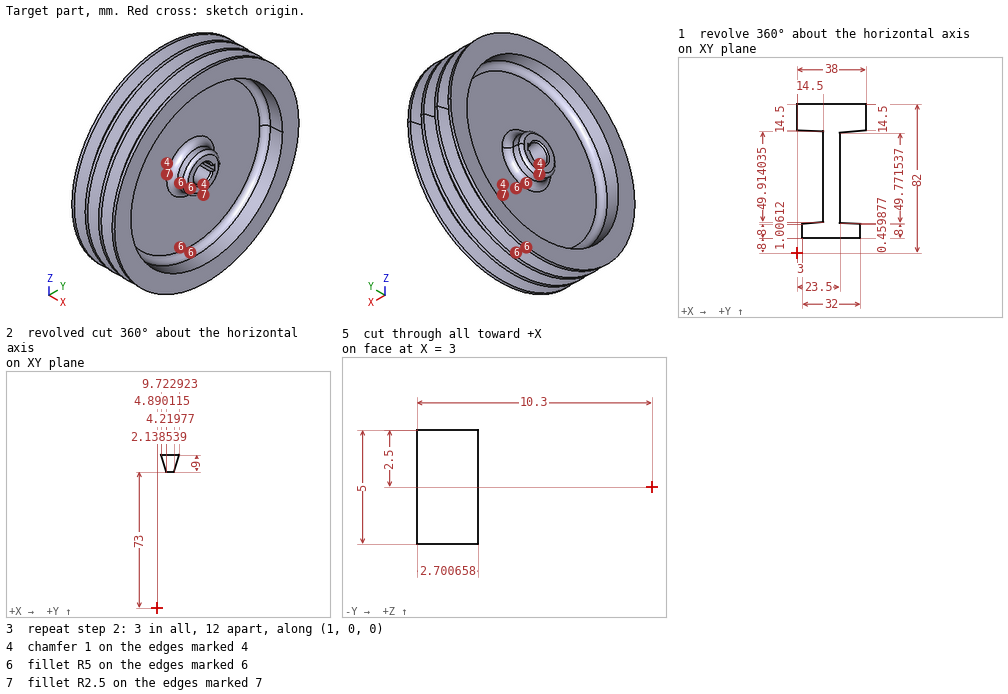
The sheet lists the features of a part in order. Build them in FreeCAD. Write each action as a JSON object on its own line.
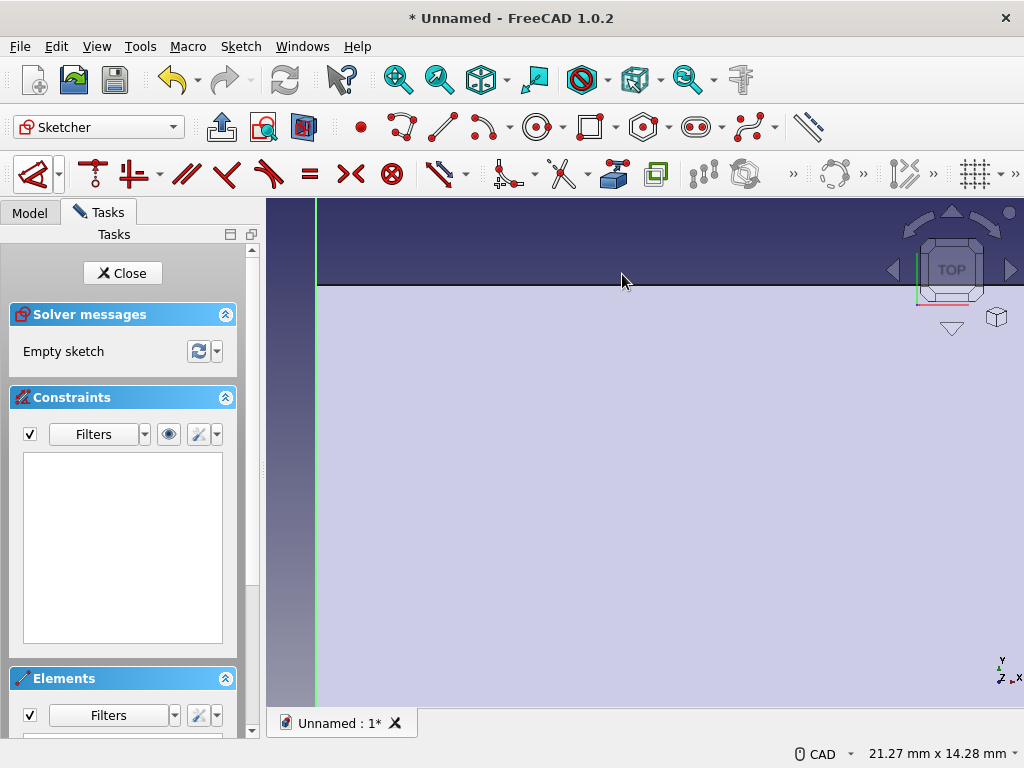
{"action": "left_click", "coordinate": [402, 128]}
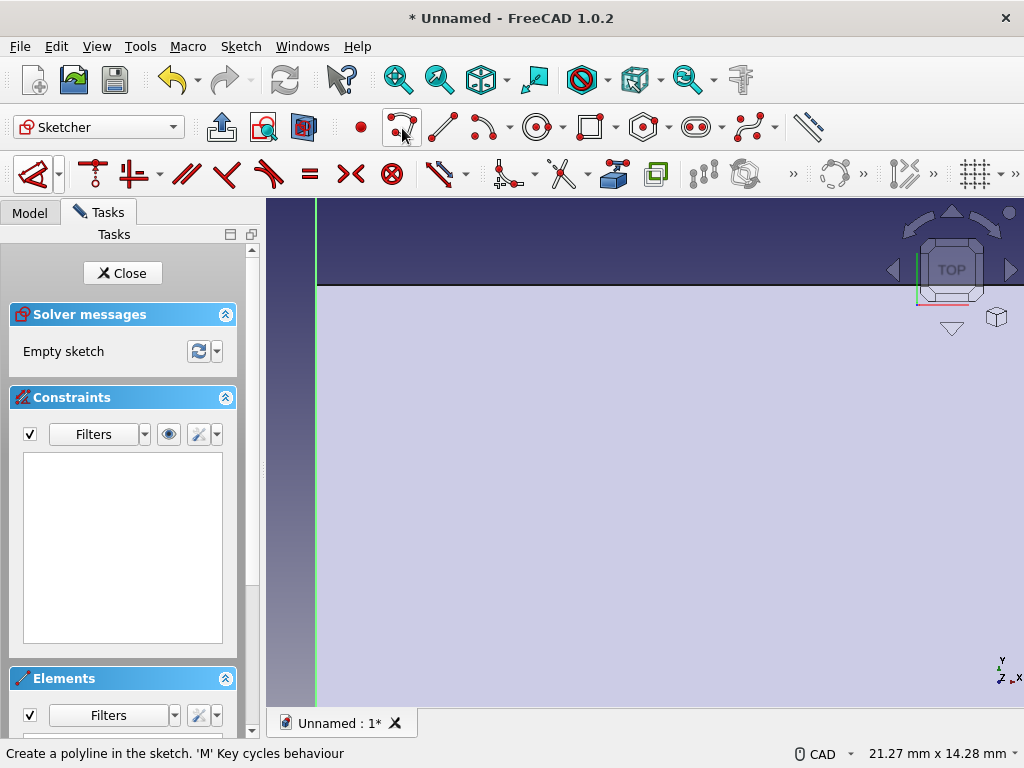
{"action": "left_click", "coordinate": [490, 605]}
{"action": "left_click", "coordinate": [640, 605]}
{"action": "left_click", "coordinate": [739, 285]}
{"action": "left_click", "coordinate": [392, 285]}
{"action": "left_click", "coordinate": [490, 606]}
{"action": "key", "text": "Escape"}
{"action": "key", "text": "Escape"}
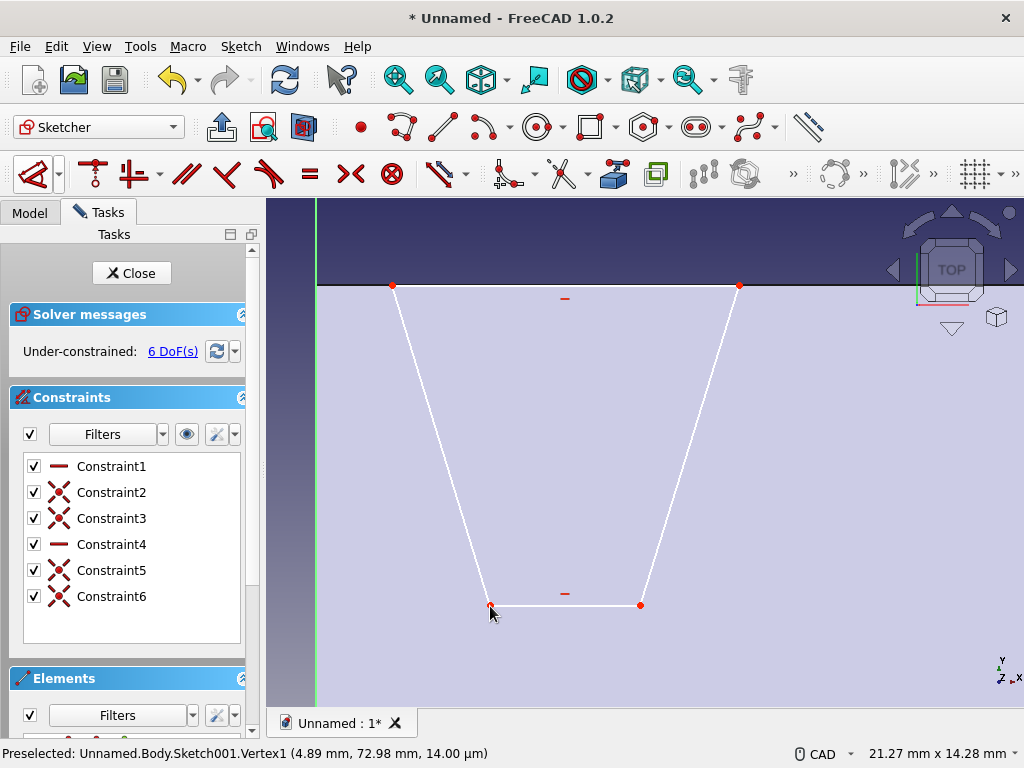
{"action": "left_click", "coordinate": [670, 510]}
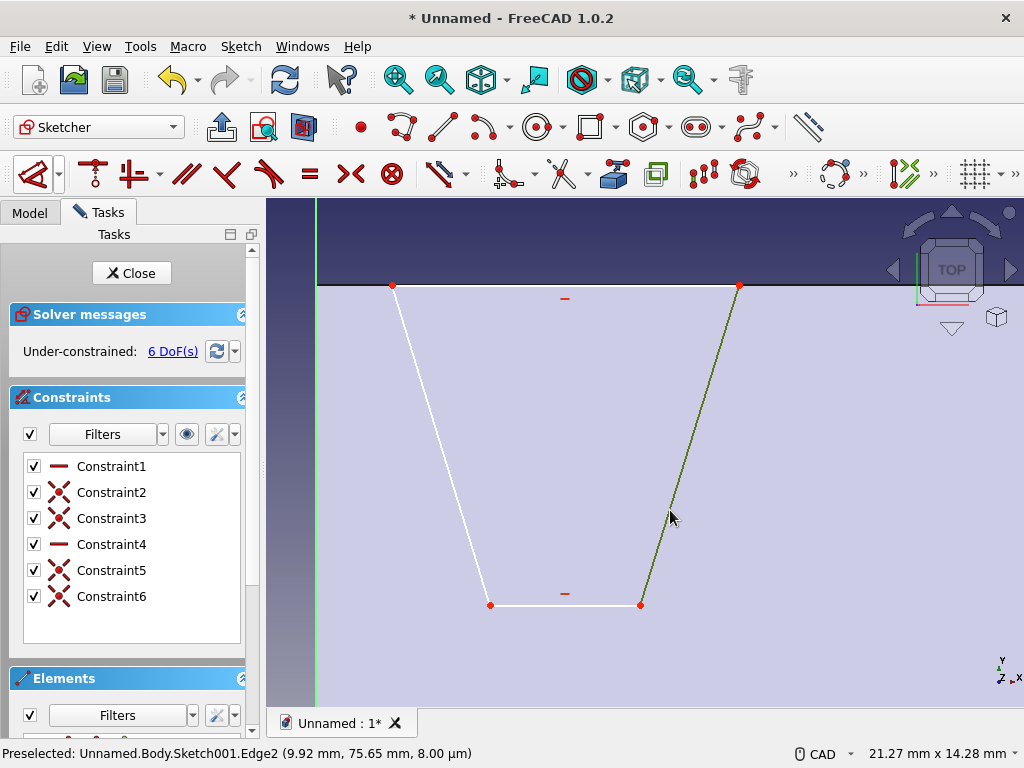
{"action": "key", "text": "i"}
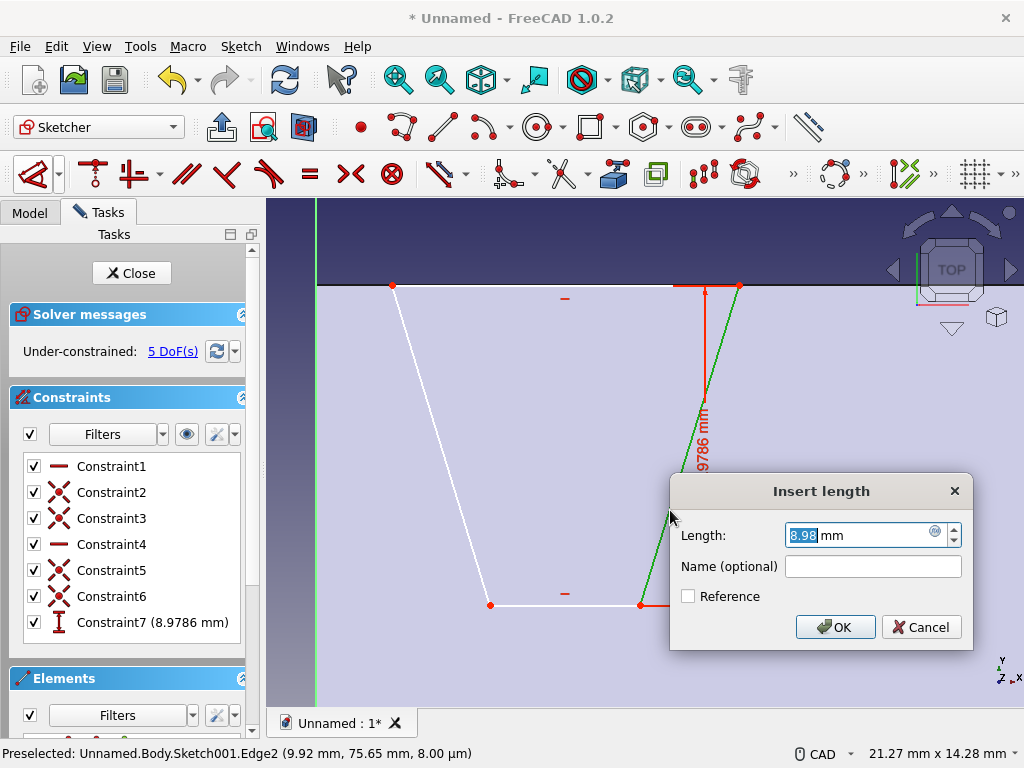
{"action": "type", "text": "9"}
{"action": "key", "text": "Return"}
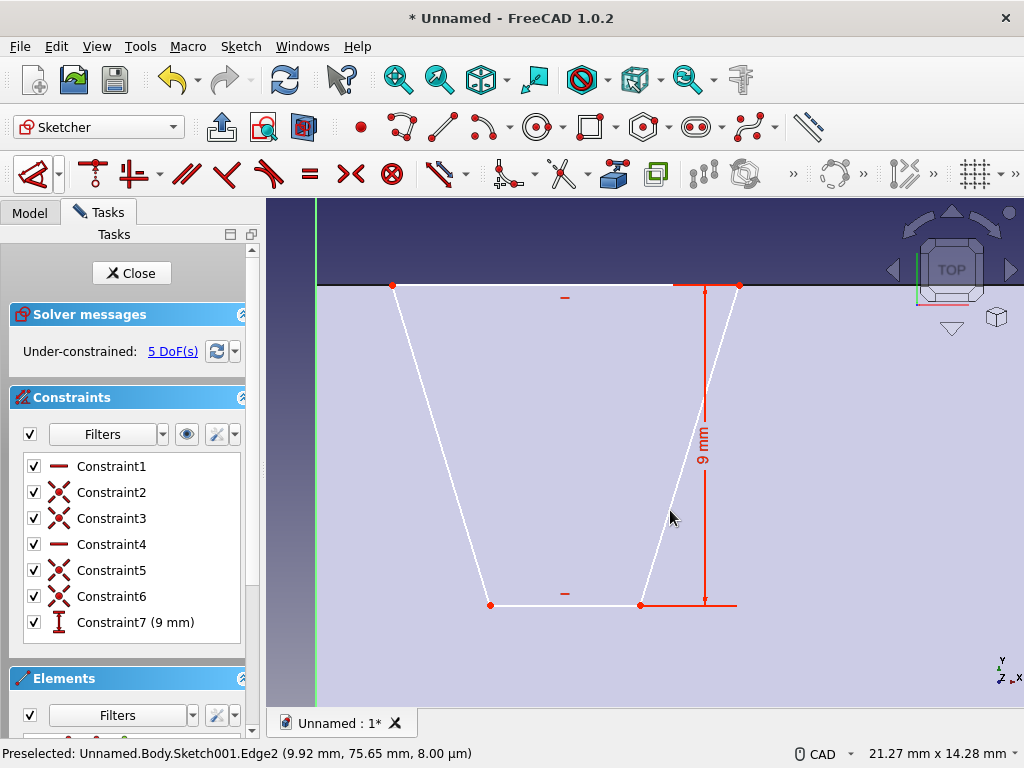
{"action": "left_click", "coordinate": [490, 606]}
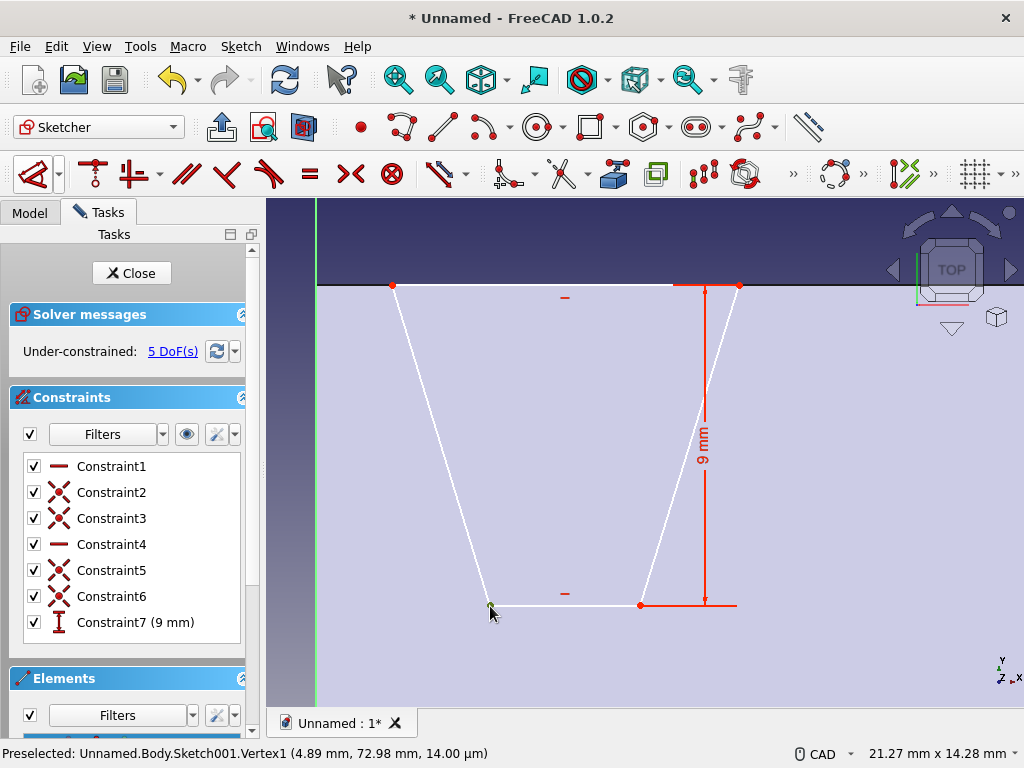
{"action": "key", "text": "i"}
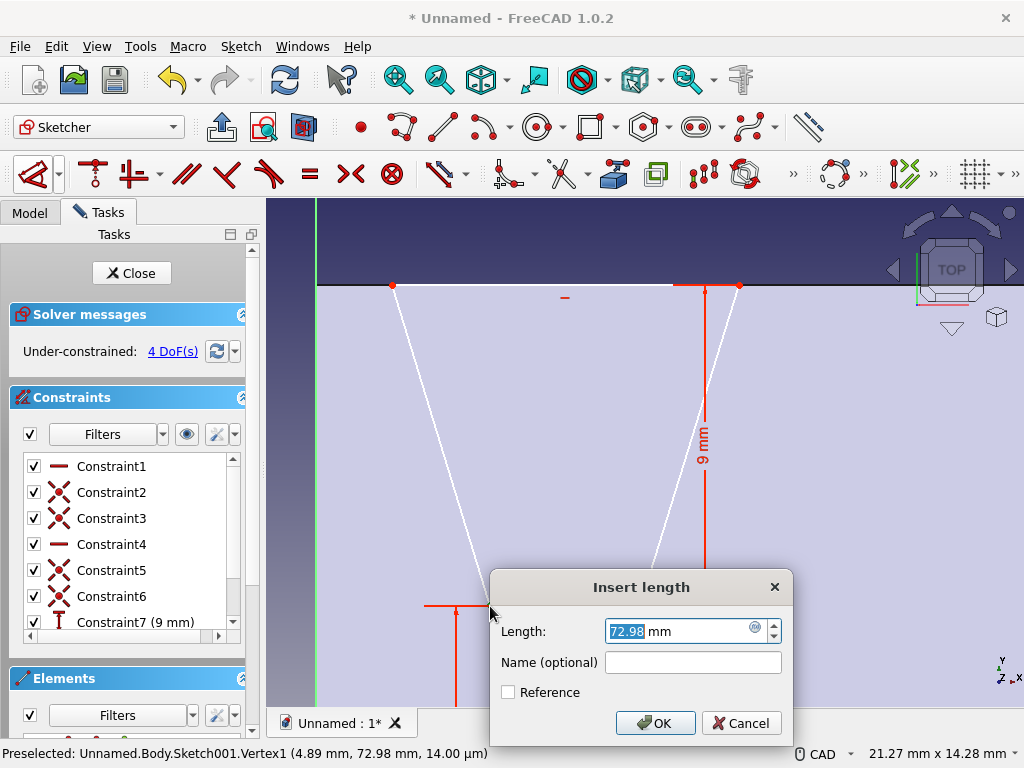
{"action": "type", "text": "73"}
{"action": "key", "text": "Return"}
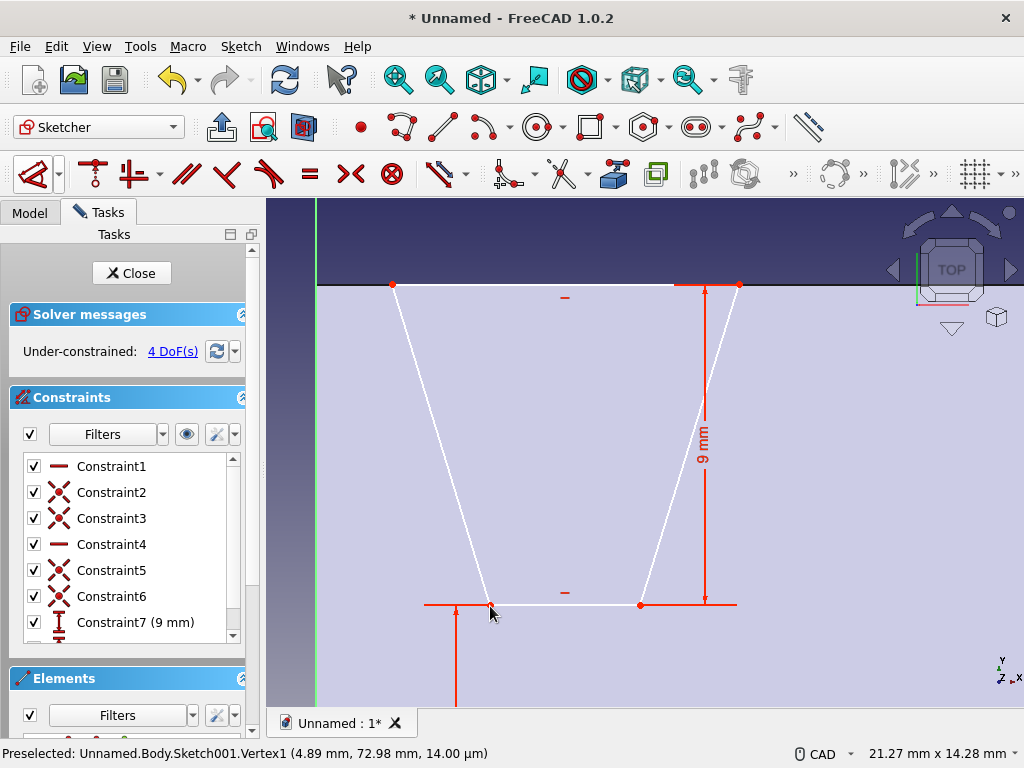
{"action": "left_click", "coordinate": [535, 605]}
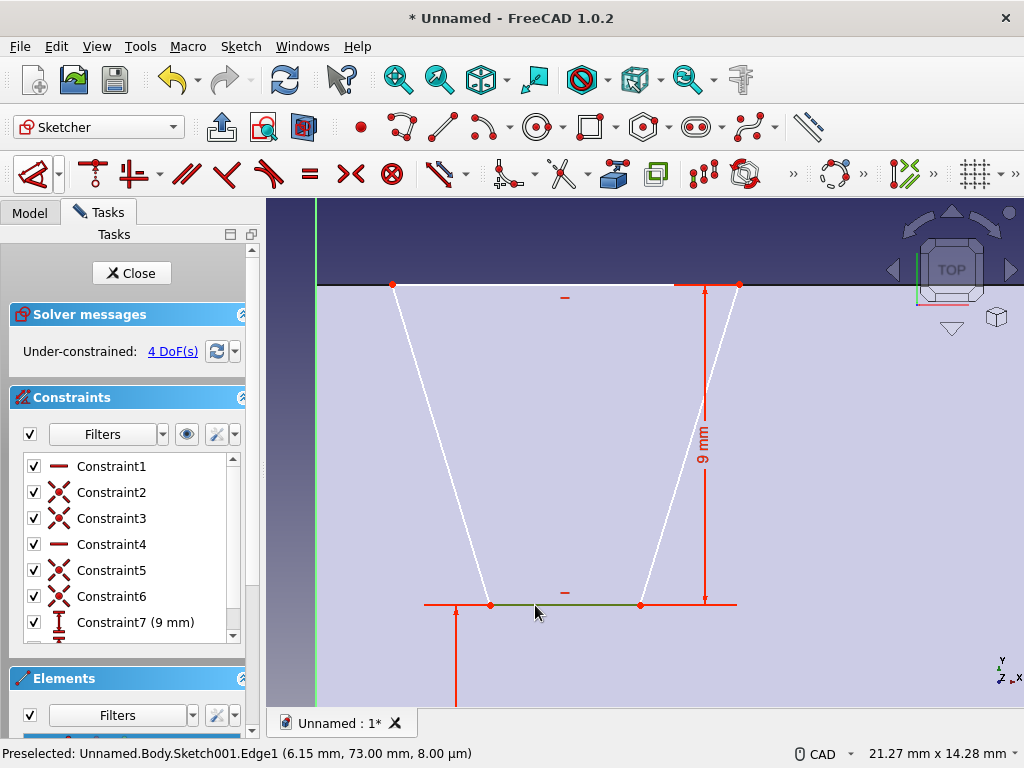
{"action": "key", "text": "l"}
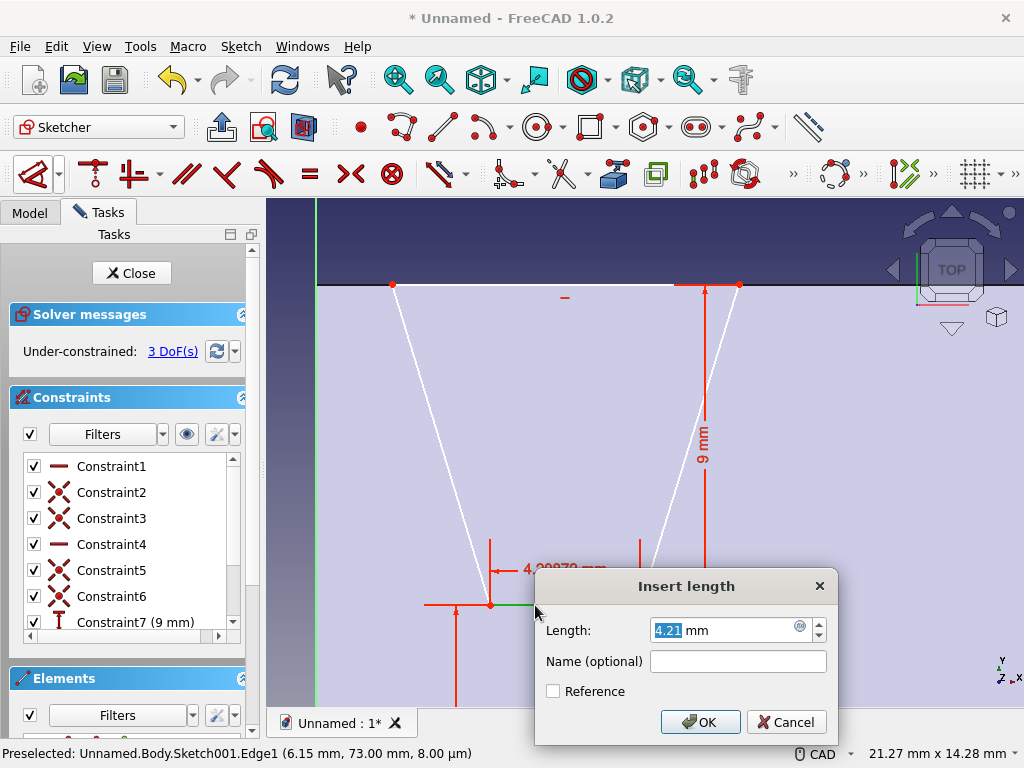
{"action": "type", "text": "4.21977"}
{"action": "key", "text": "Return"}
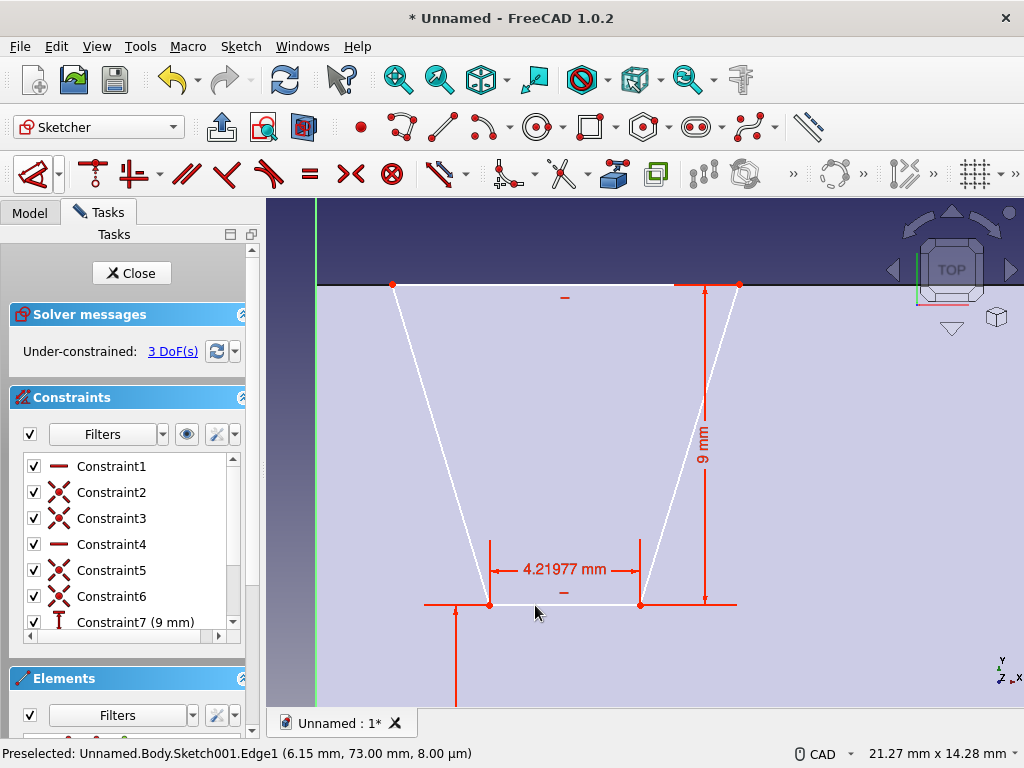
{"action": "left_click", "coordinate": [635, 285]}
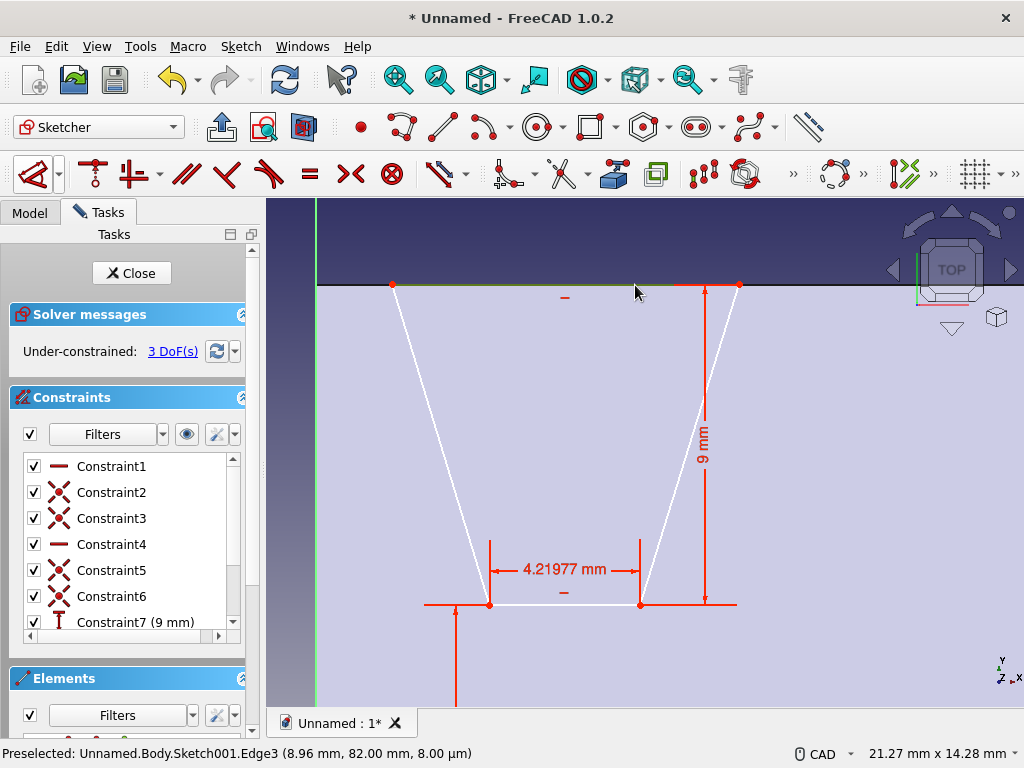
{"action": "key", "text": "l"}